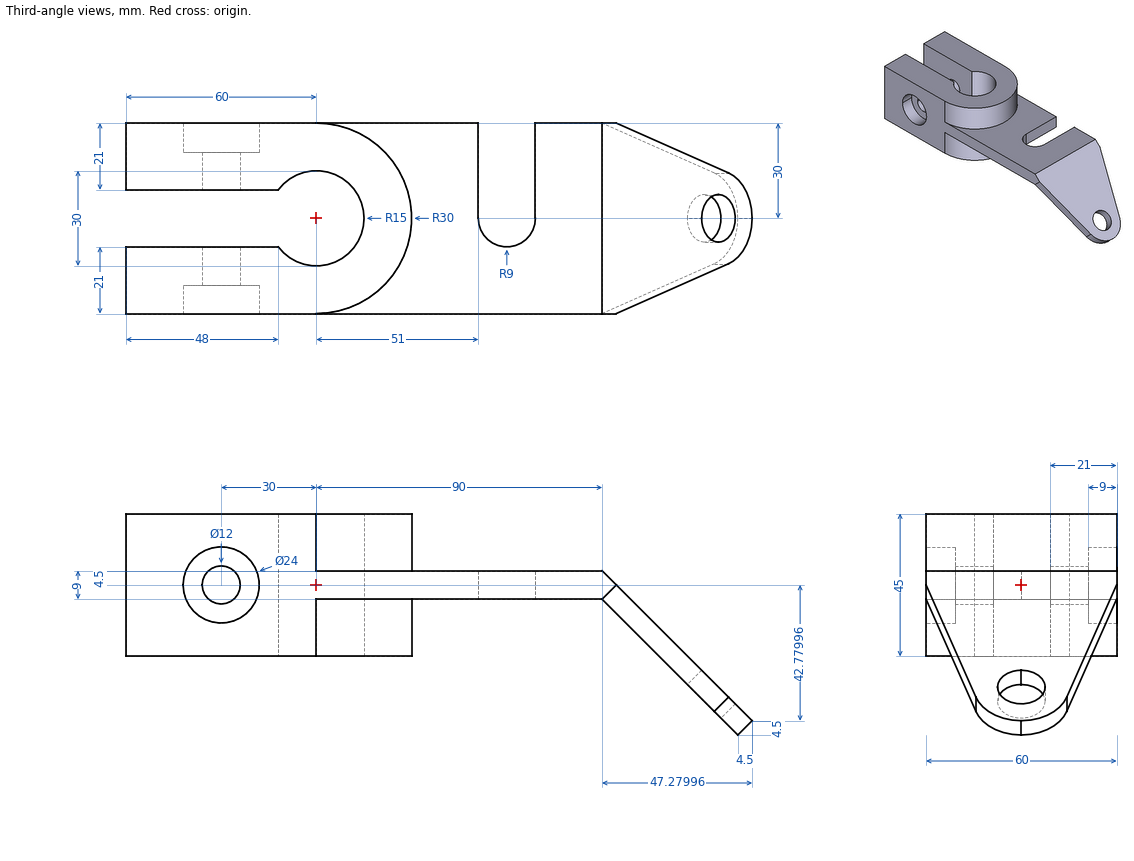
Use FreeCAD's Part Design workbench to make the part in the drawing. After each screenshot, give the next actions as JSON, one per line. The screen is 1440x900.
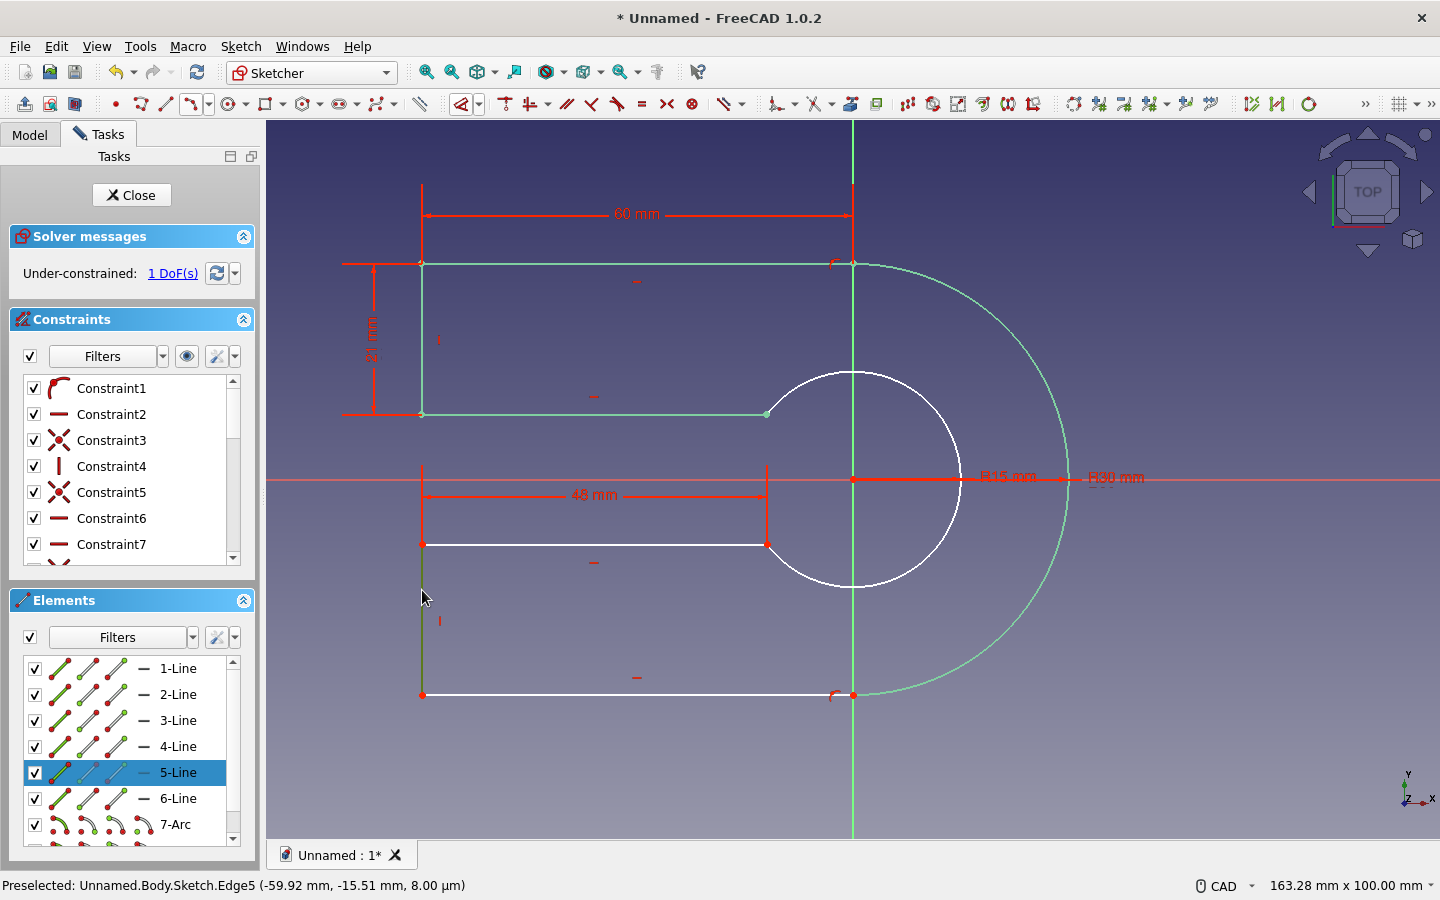
{"action": "left_click", "coordinate": [478, 104]}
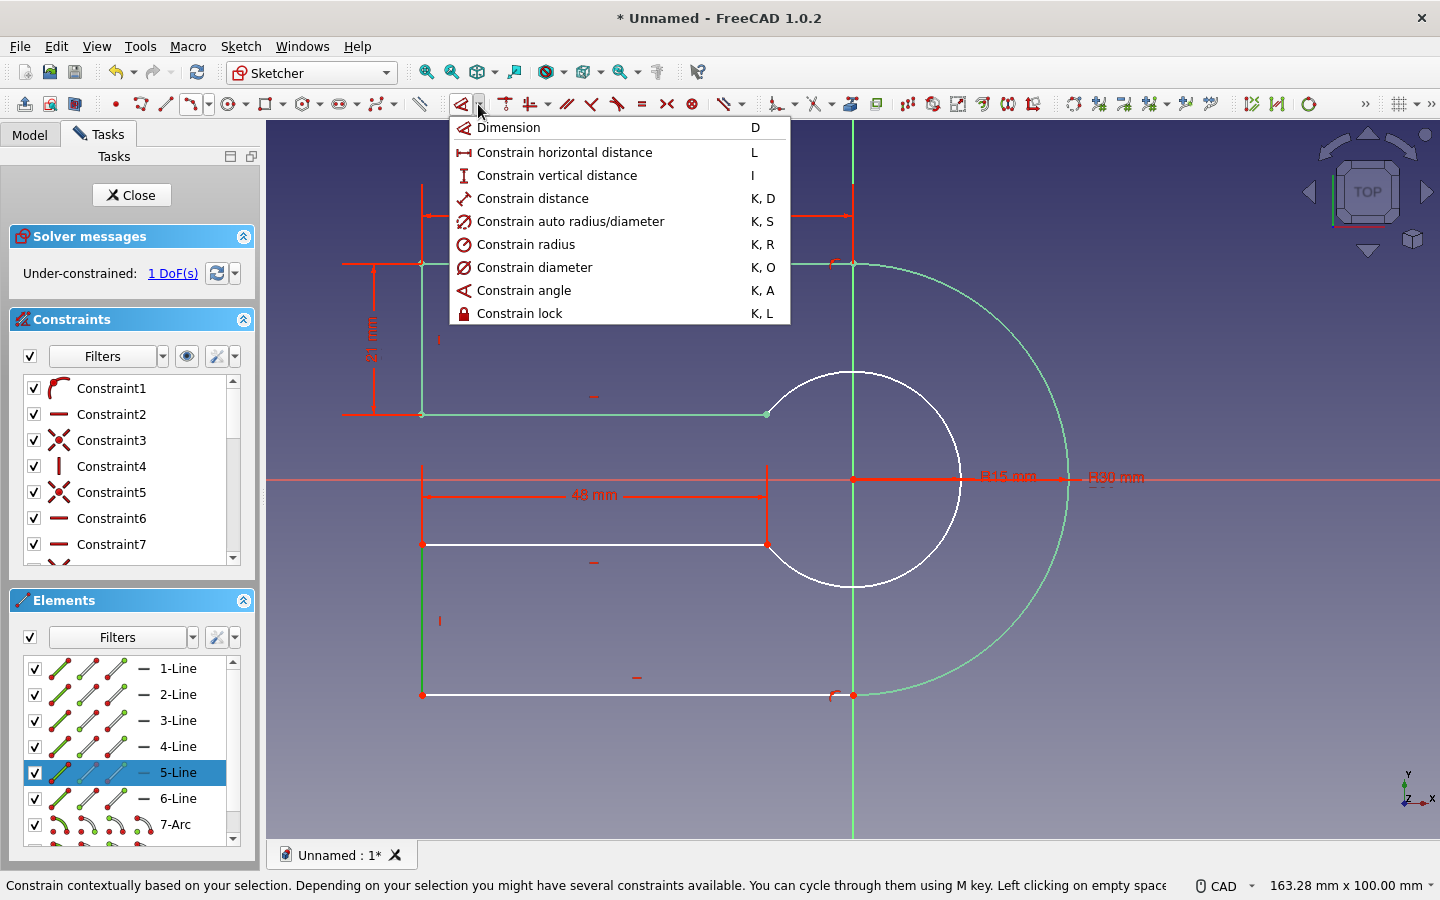
{"action": "left_click", "coordinate": [620, 176]}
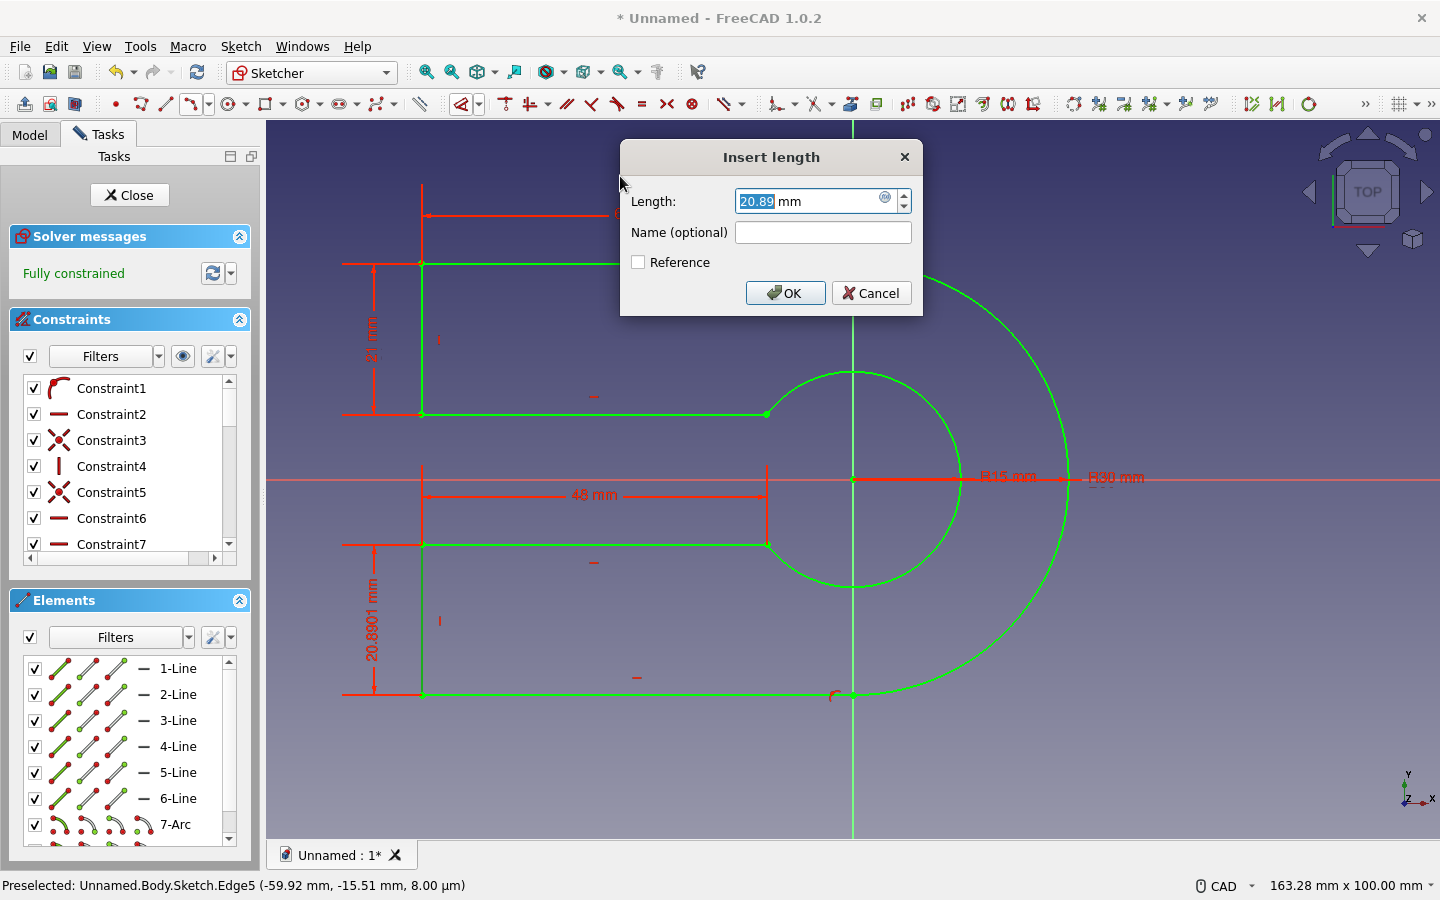
{"action": "type", "text": "21"}
{"action": "key", "text": "Return"}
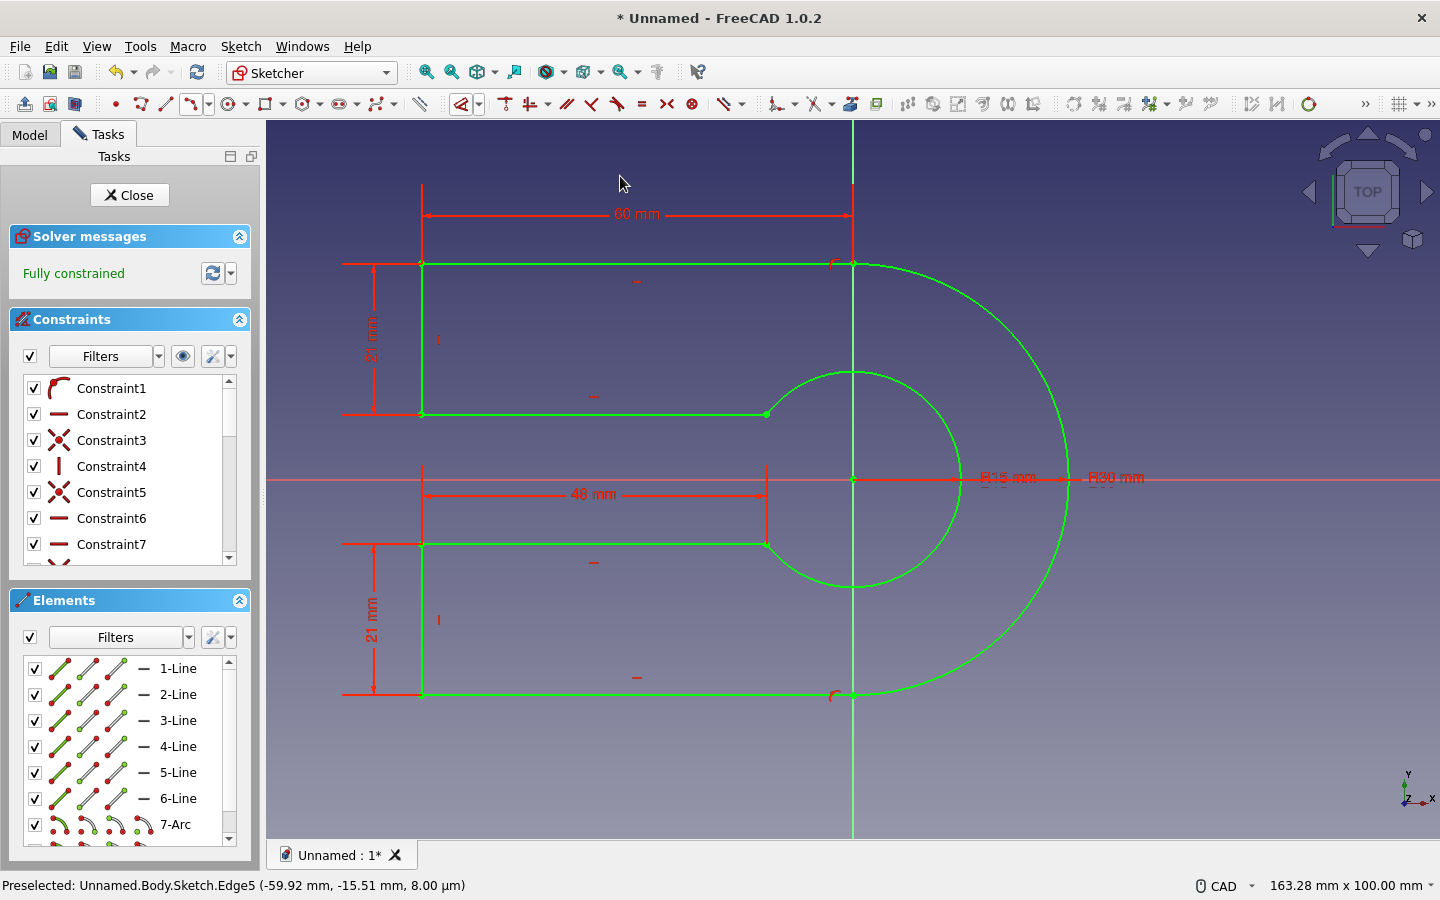
{"action": "left_click", "coordinate": [130, 195]}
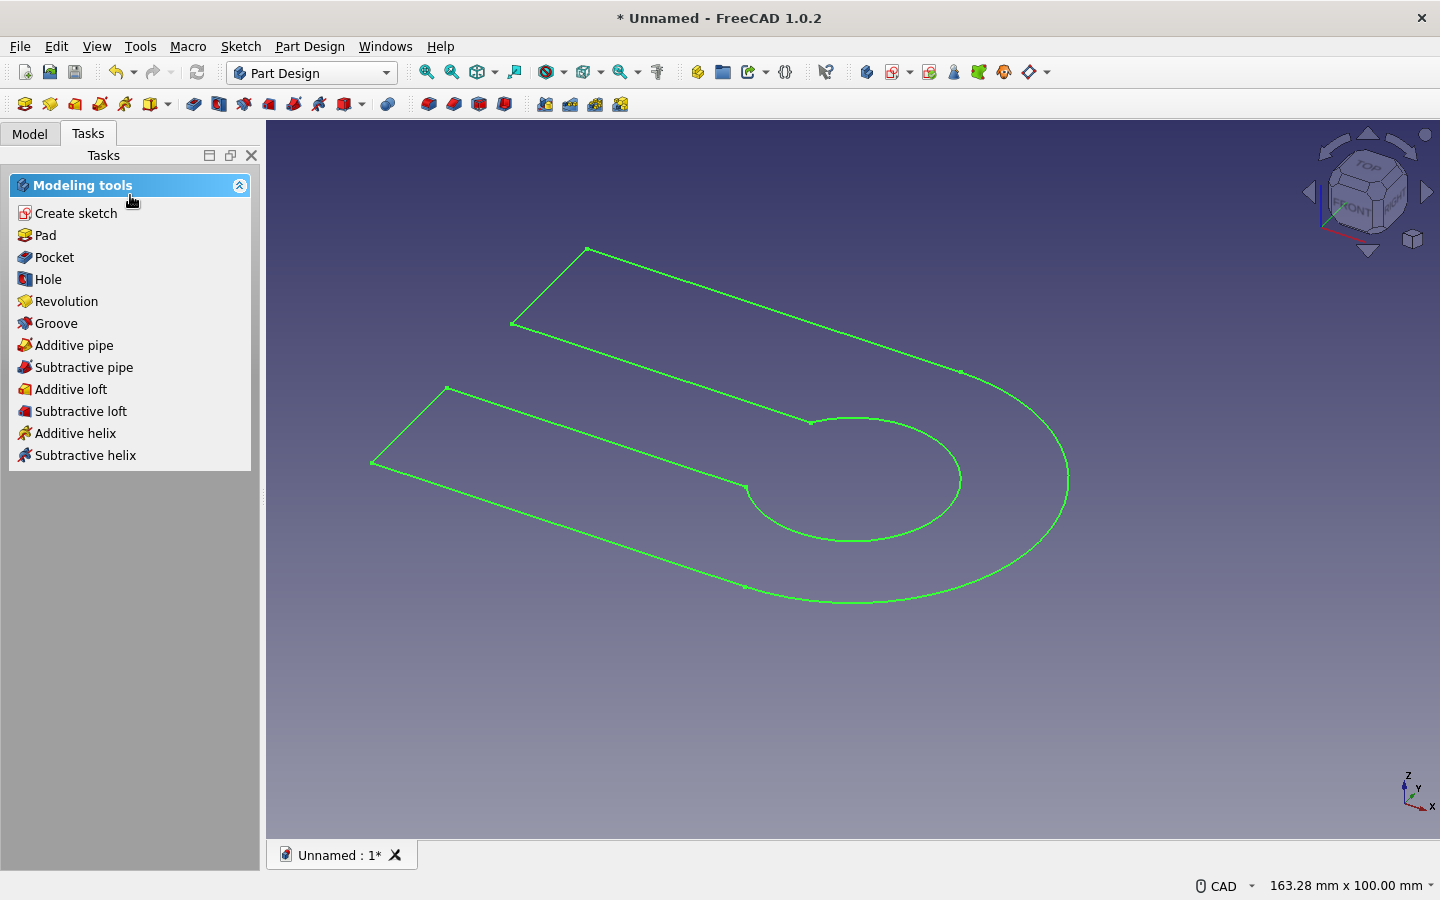
{"action": "left_click", "coordinate": [25, 104]}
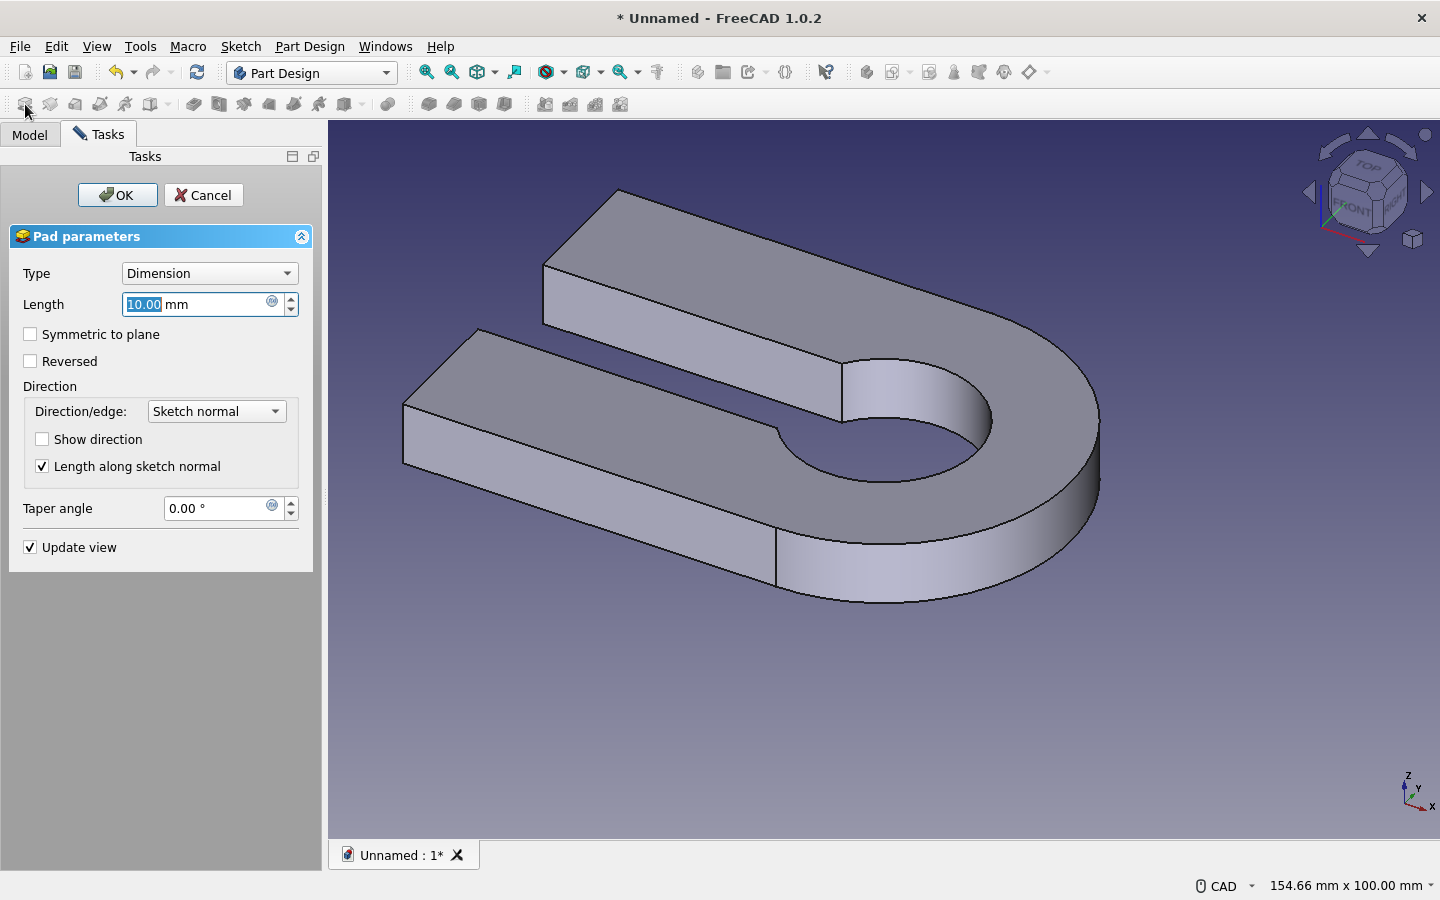
{"action": "type", "text": "45"}
{"action": "key", "text": "Tab"}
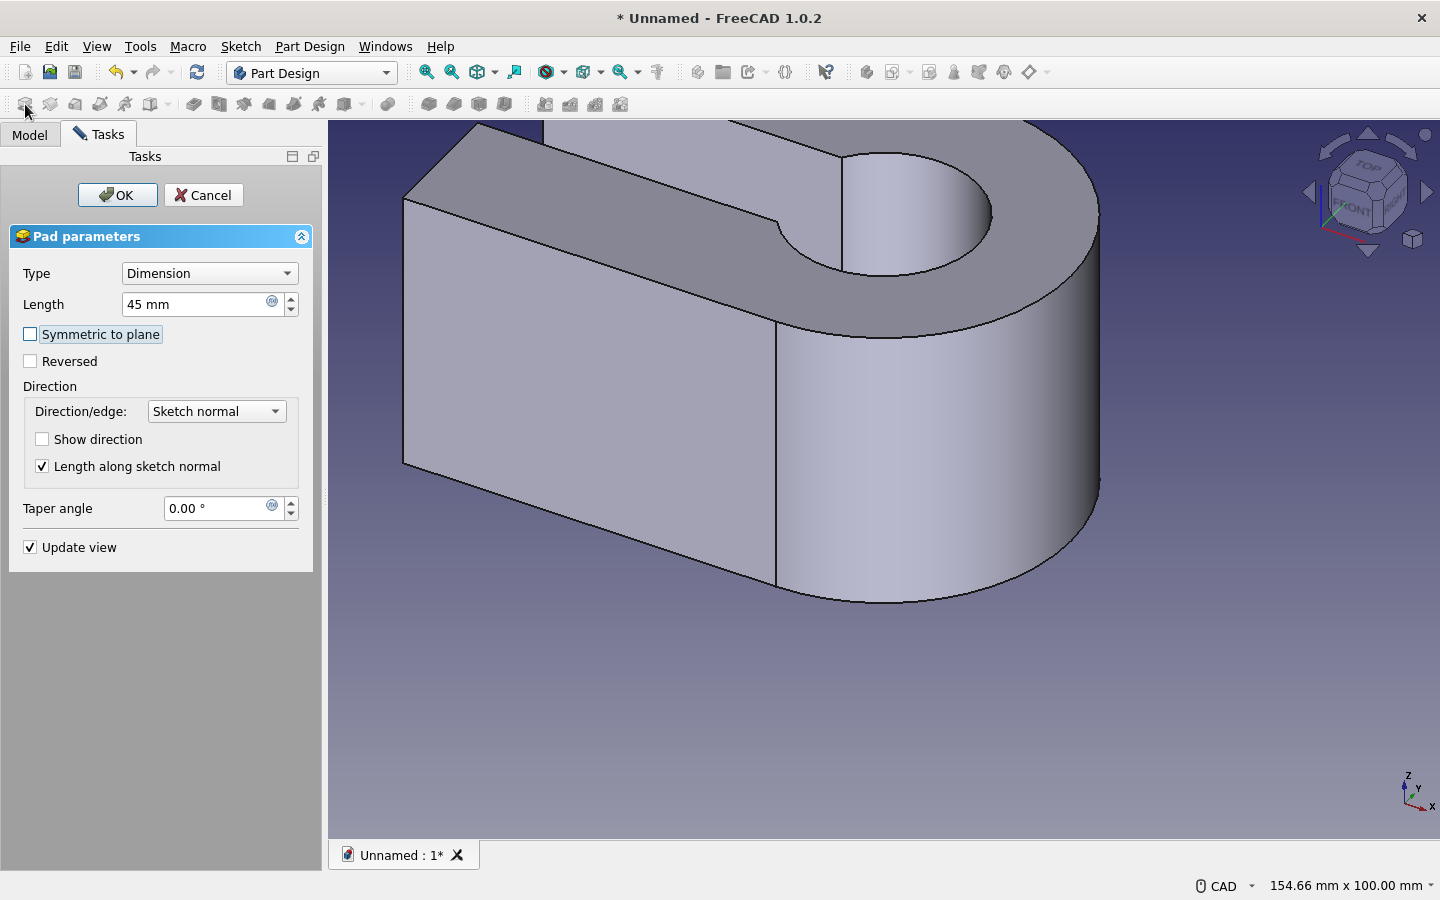
{"action": "left_click", "coordinate": [31, 334]}